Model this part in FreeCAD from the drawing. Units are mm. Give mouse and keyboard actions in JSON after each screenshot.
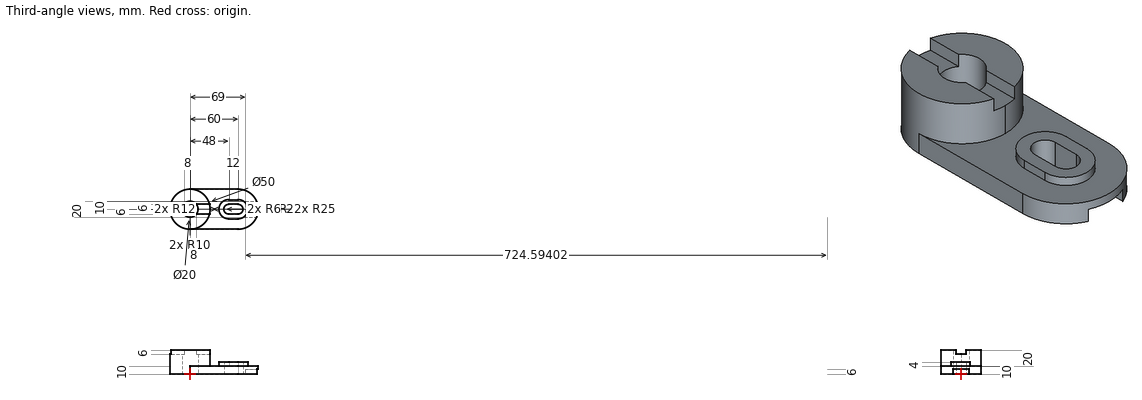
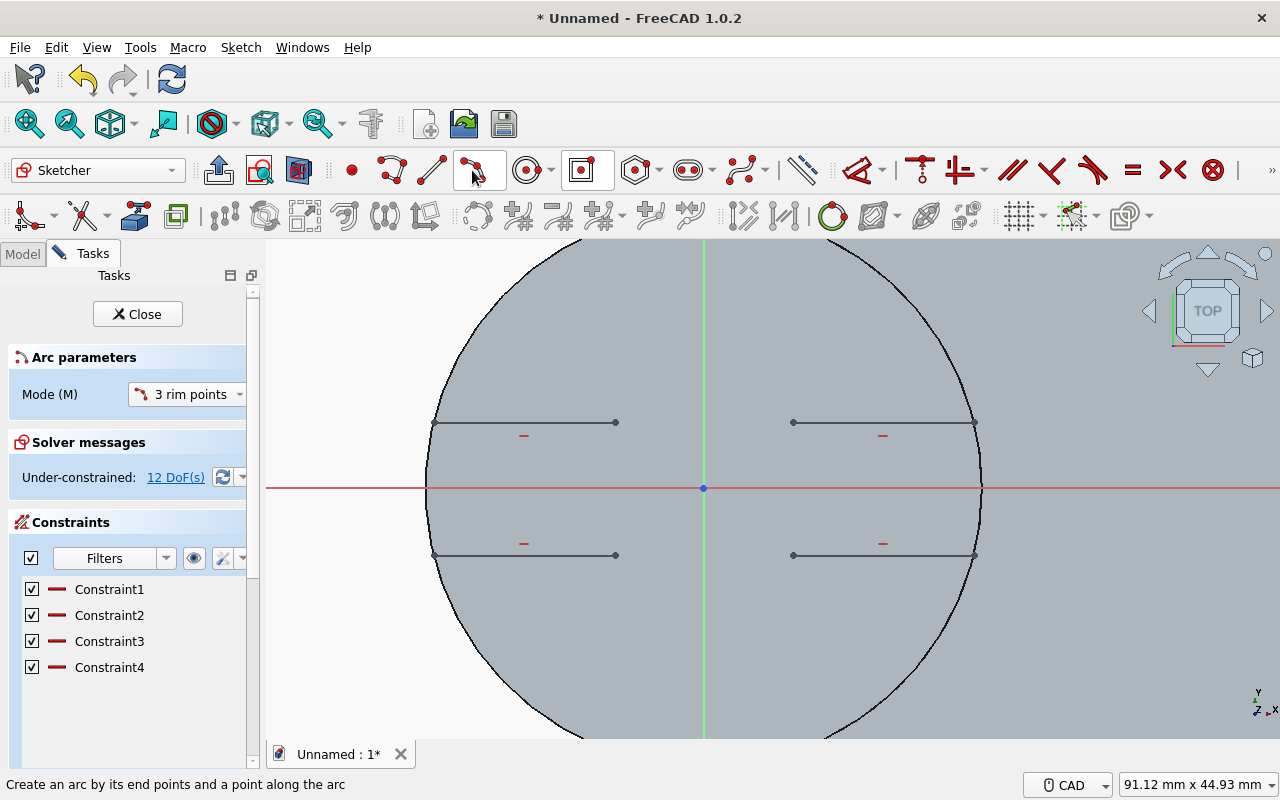
{"action": "left_click", "coordinate": [793, 423]}
{"action": "left_click", "coordinate": [615, 423]}
{"action": "left_click", "coordinate": [724, 379]}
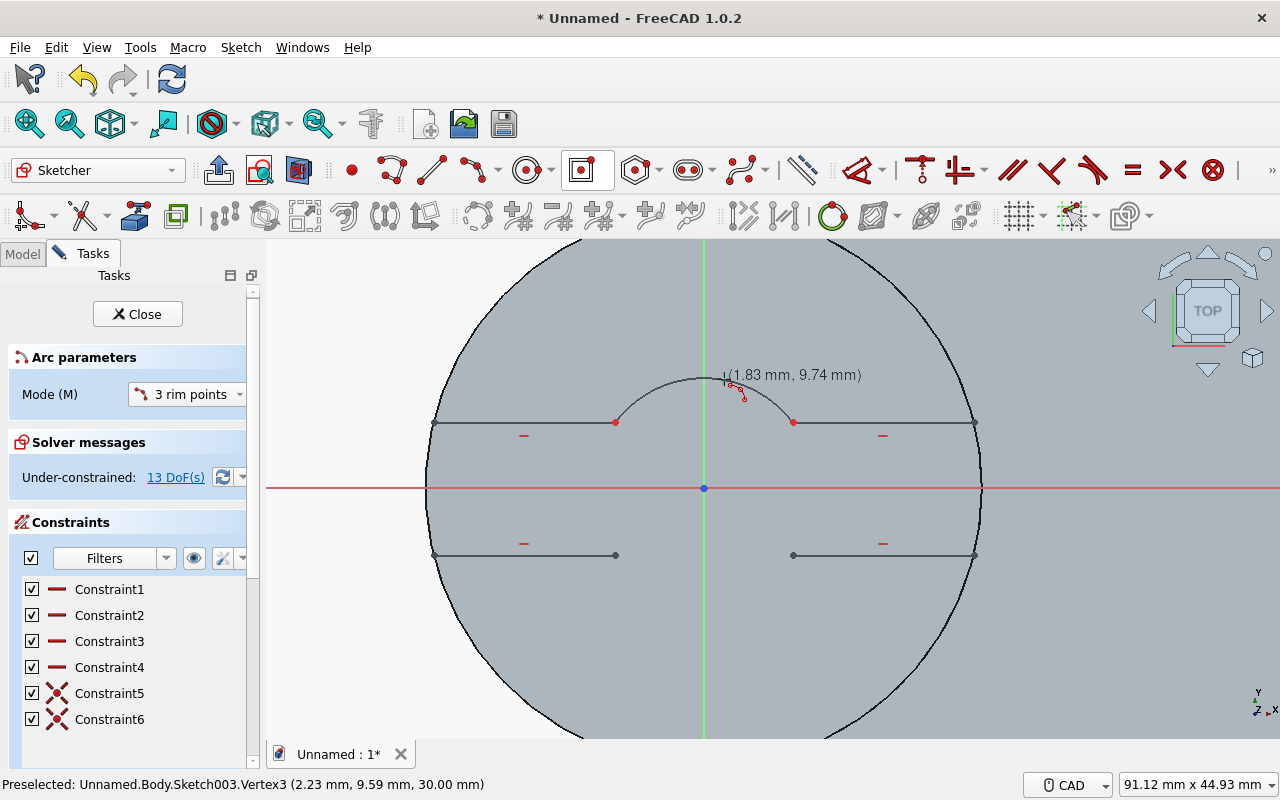
{"action": "left_click", "coordinate": [434, 423]}
{"action": "left_click", "coordinate": [434, 556]}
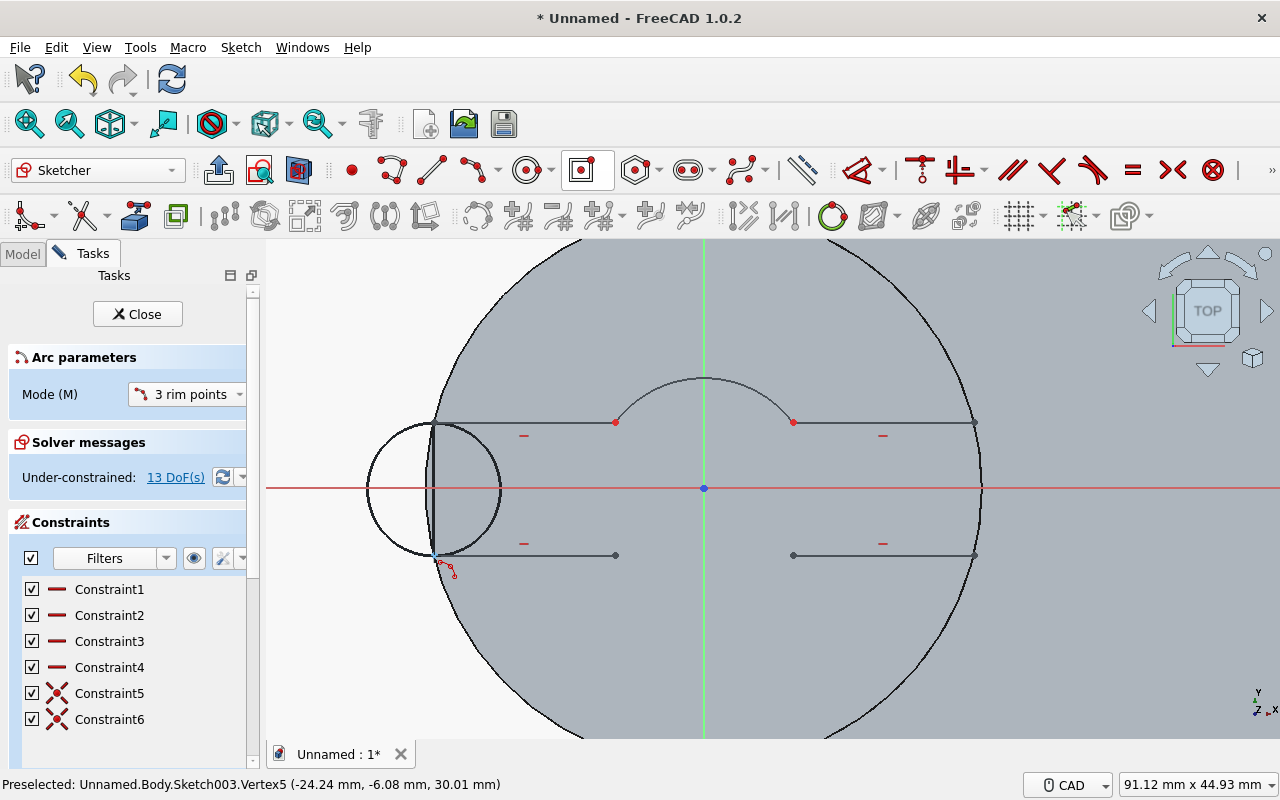
{"action": "scroll", "coordinate": [426, 475], "scroll_direction": "up", "scroll_amount": 4}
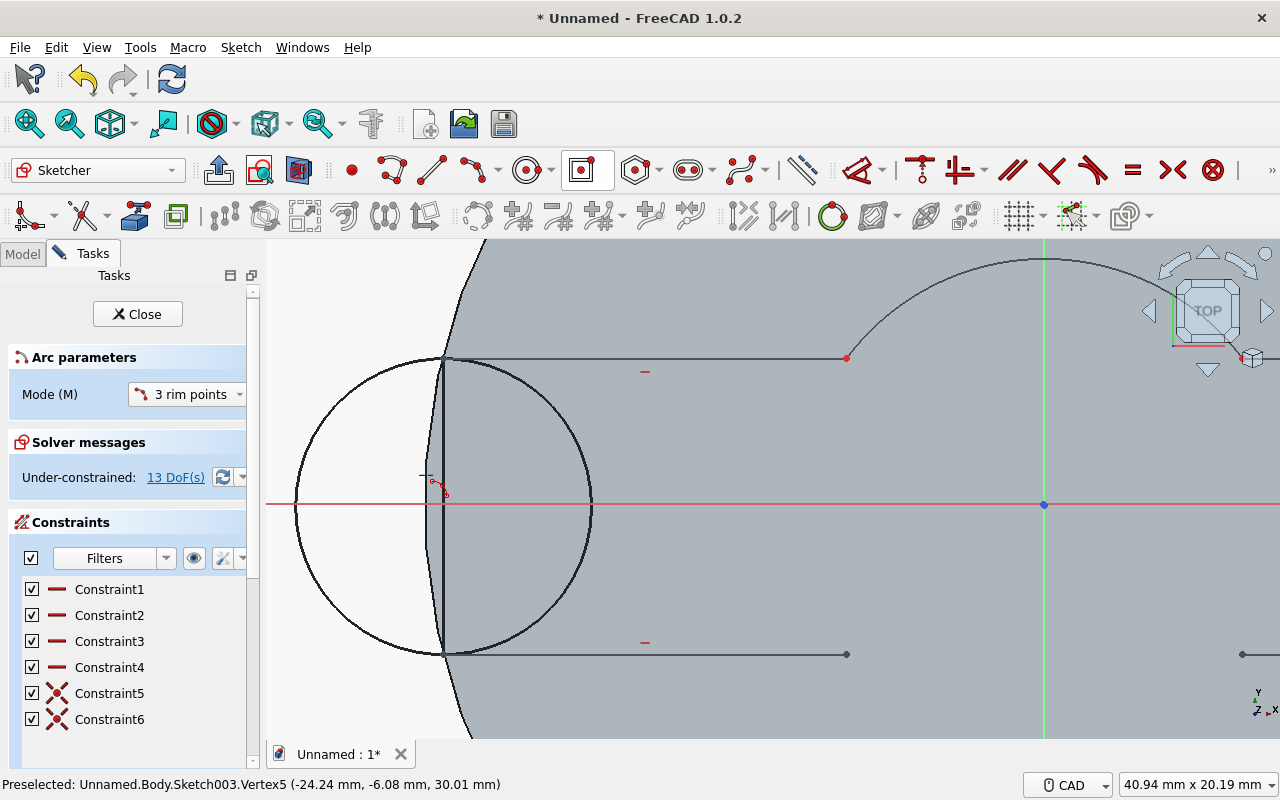
{"action": "left_click", "coordinate": [425, 474]}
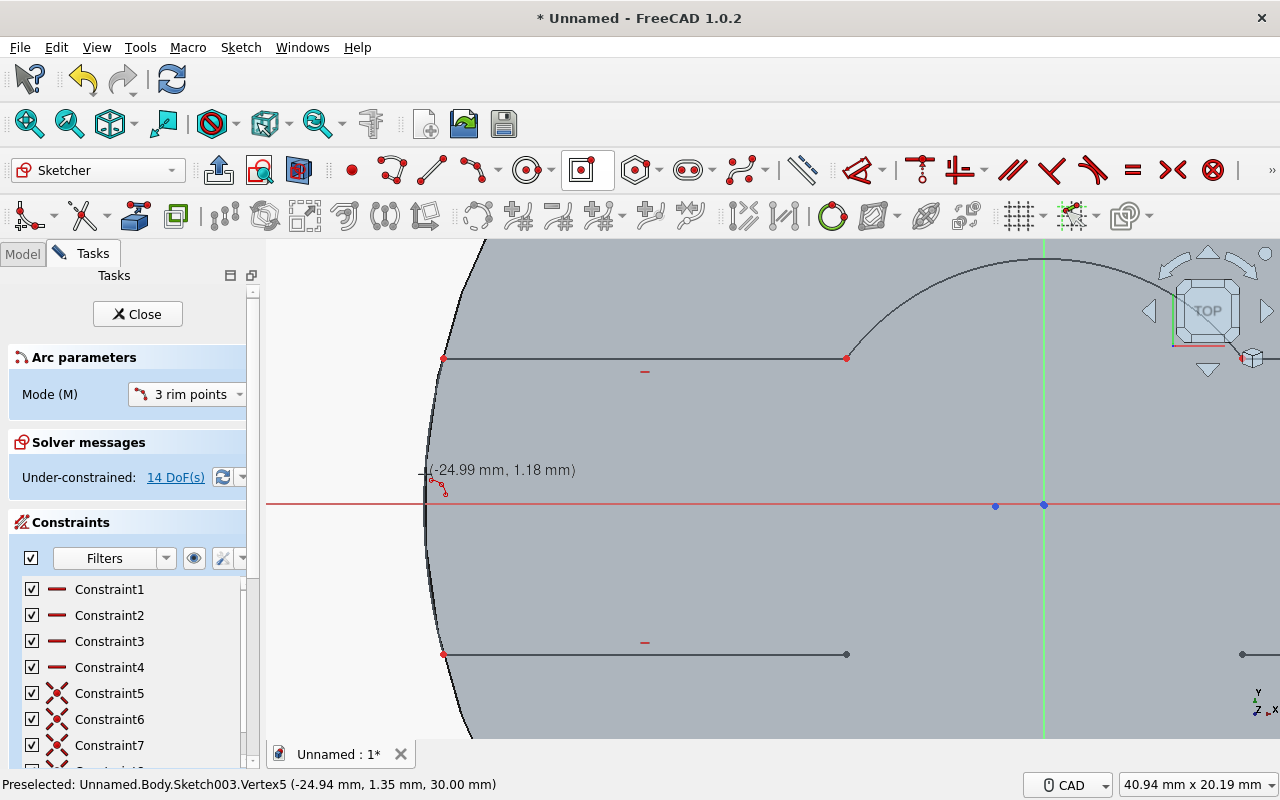
{"action": "left_click", "coordinate": [846, 655]}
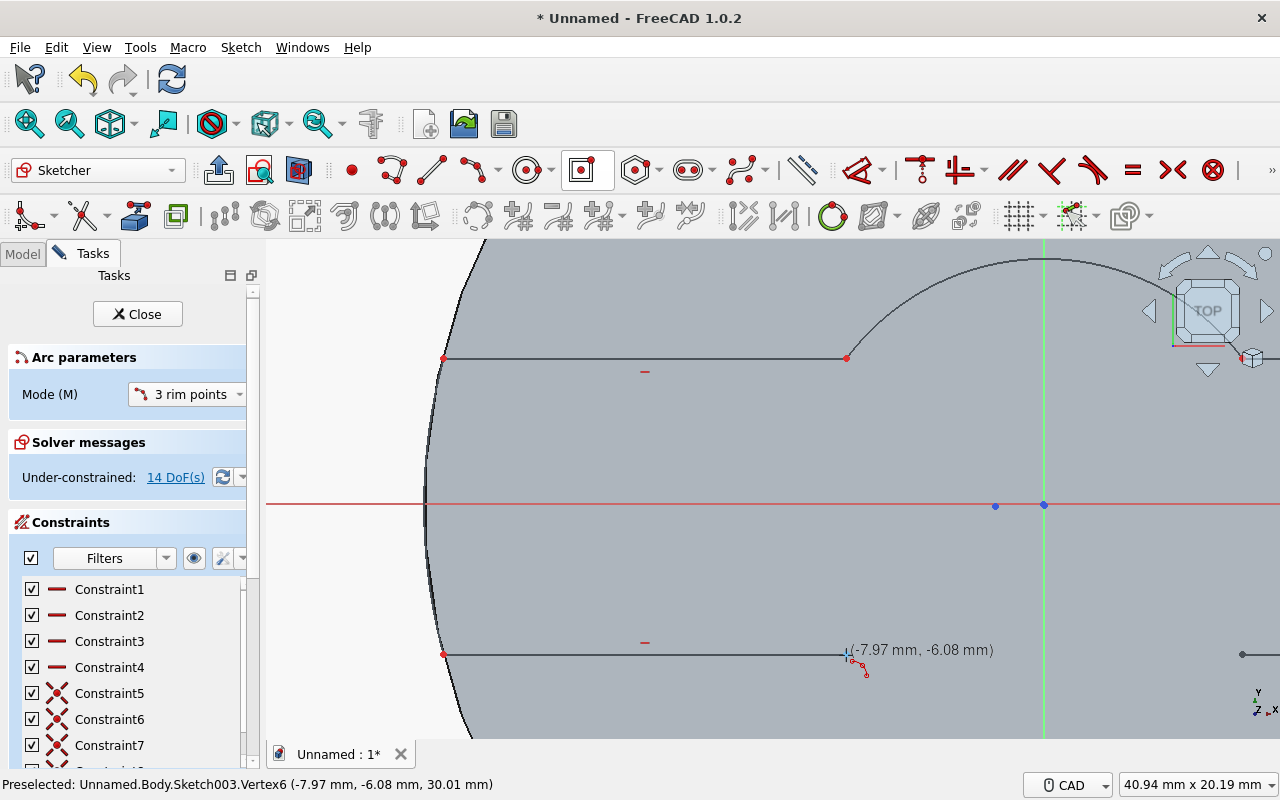
{"action": "scroll", "coordinate": [428, 477], "scroll_direction": "down", "scroll_amount": 4}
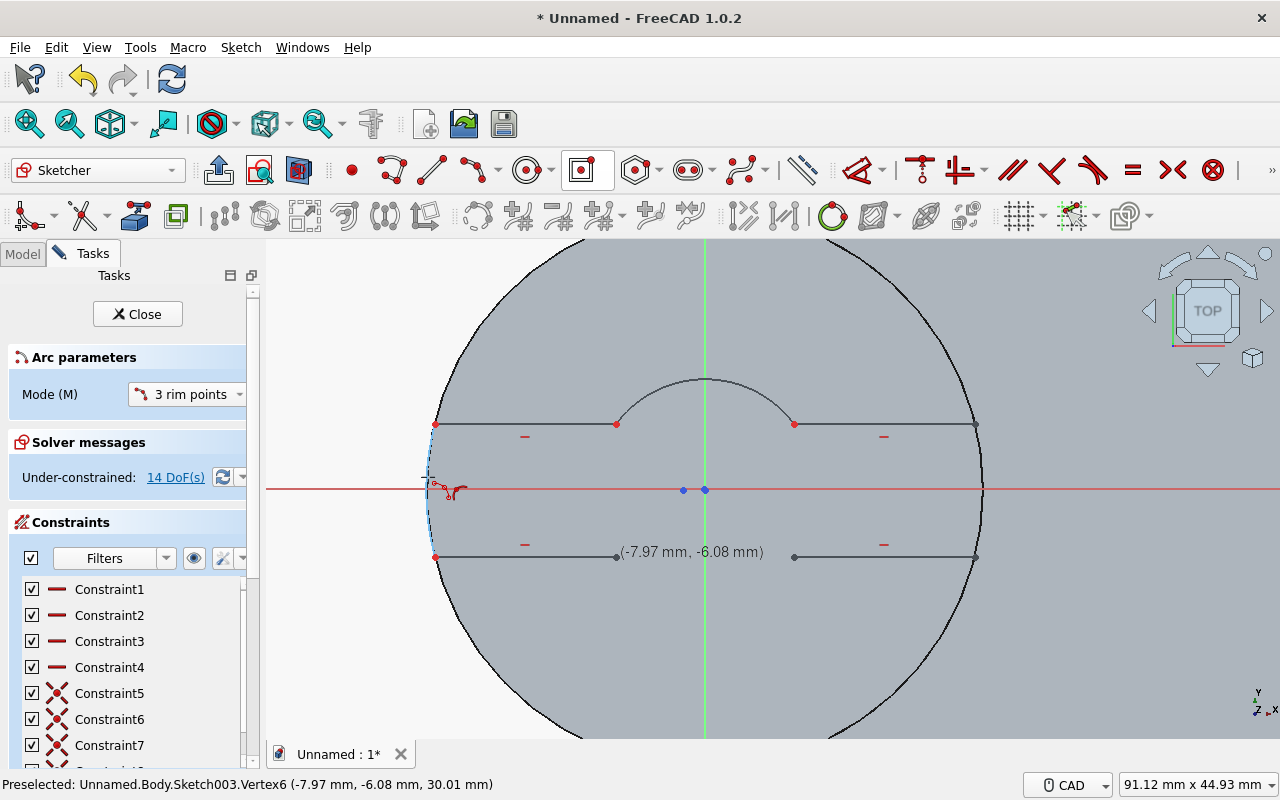
{"action": "left_click", "coordinate": [794, 557]}
{"action": "left_click", "coordinate": [684, 599]}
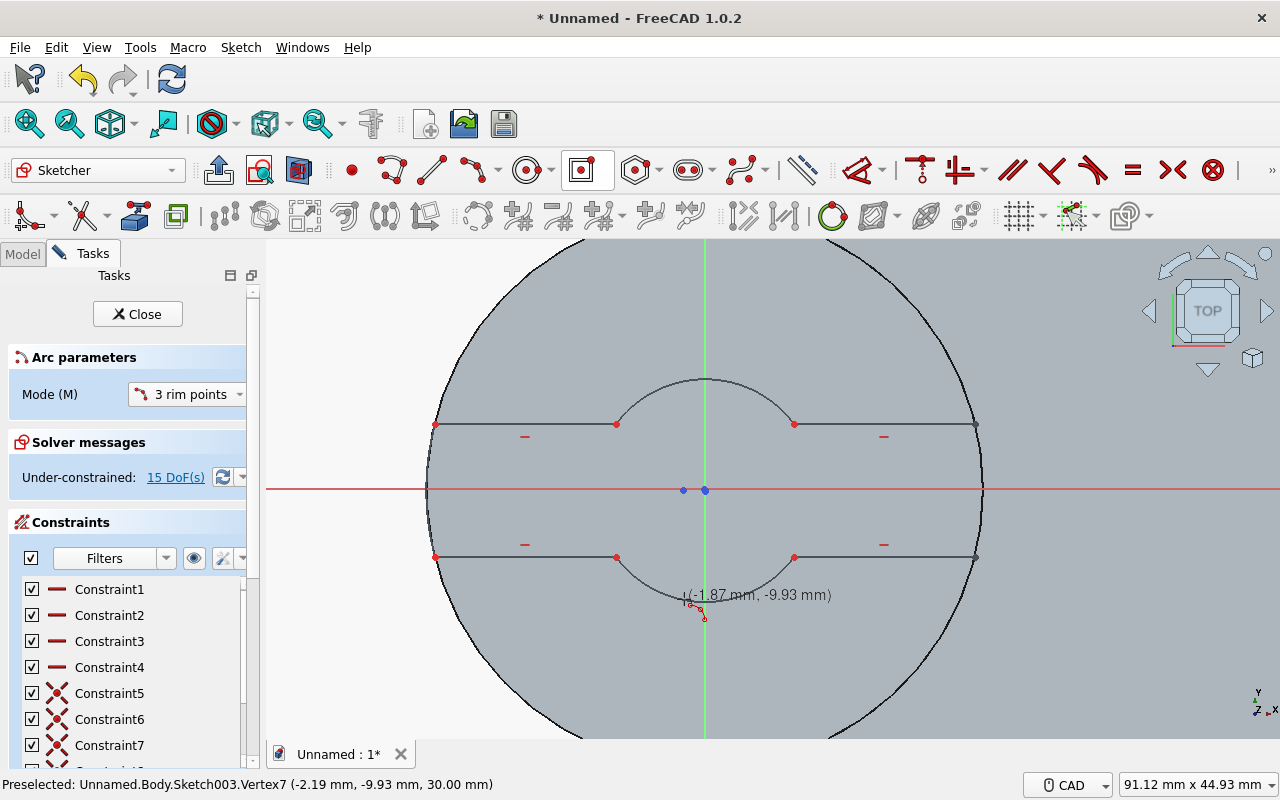
{"action": "left_click", "coordinate": [975, 557]}
{"action": "left_click", "coordinate": [975, 424]}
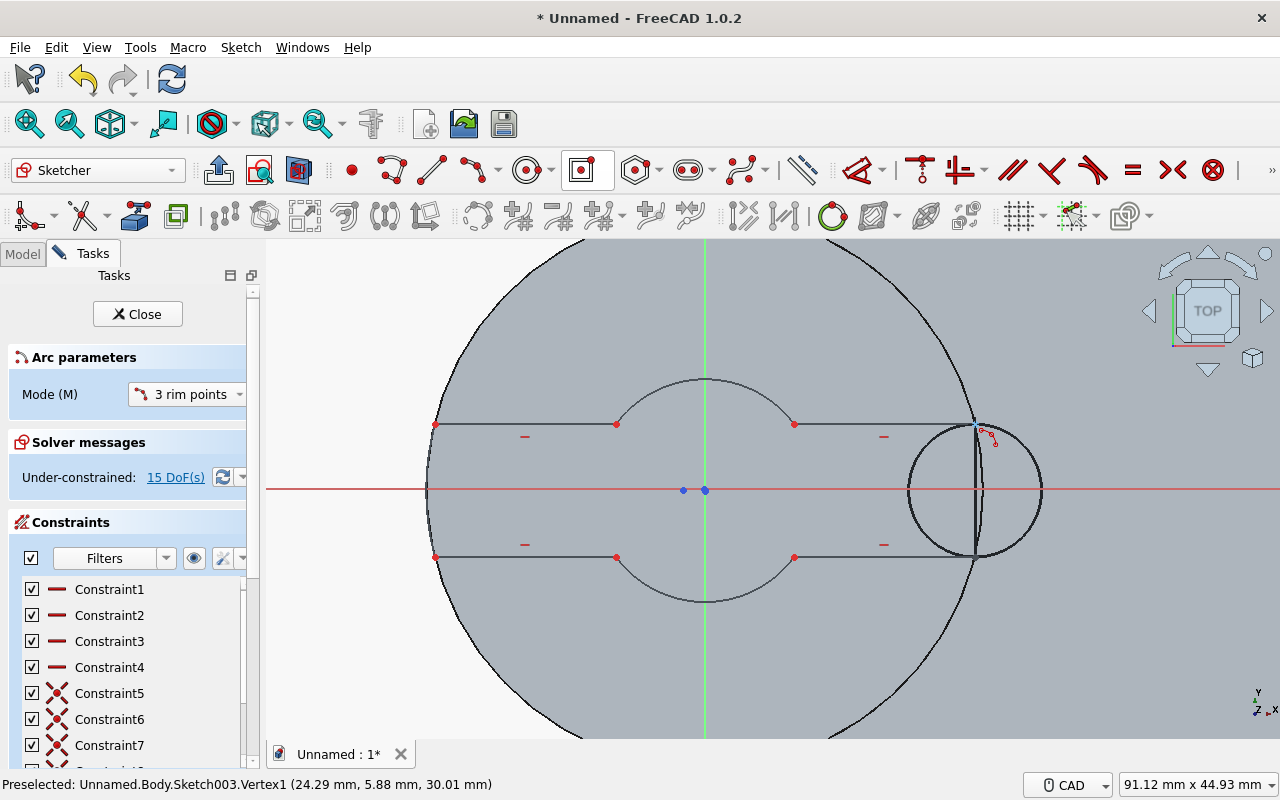
{"action": "scroll", "coordinate": [983, 503], "scroll_direction": "up", "scroll_amount": 4}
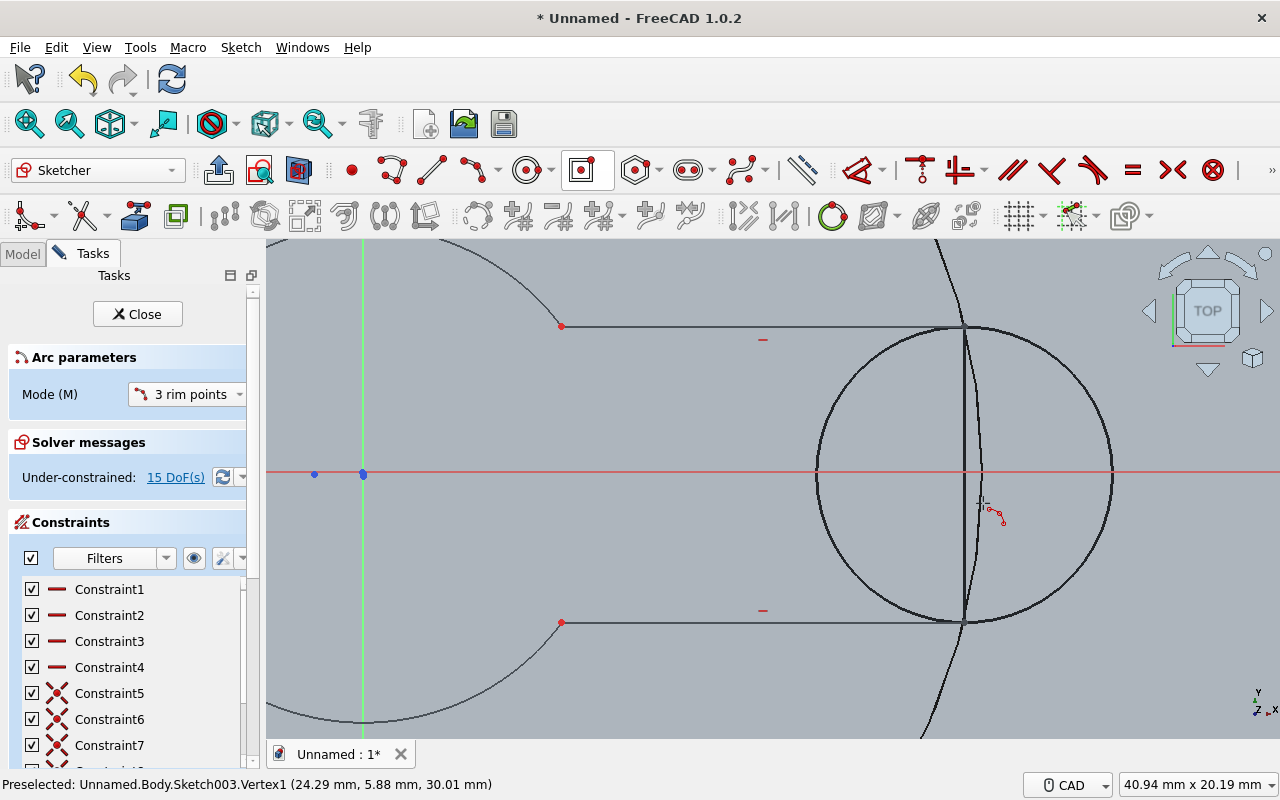
{"action": "left_click", "coordinate": [981, 502]}
{"action": "key", "text": "Escape"}